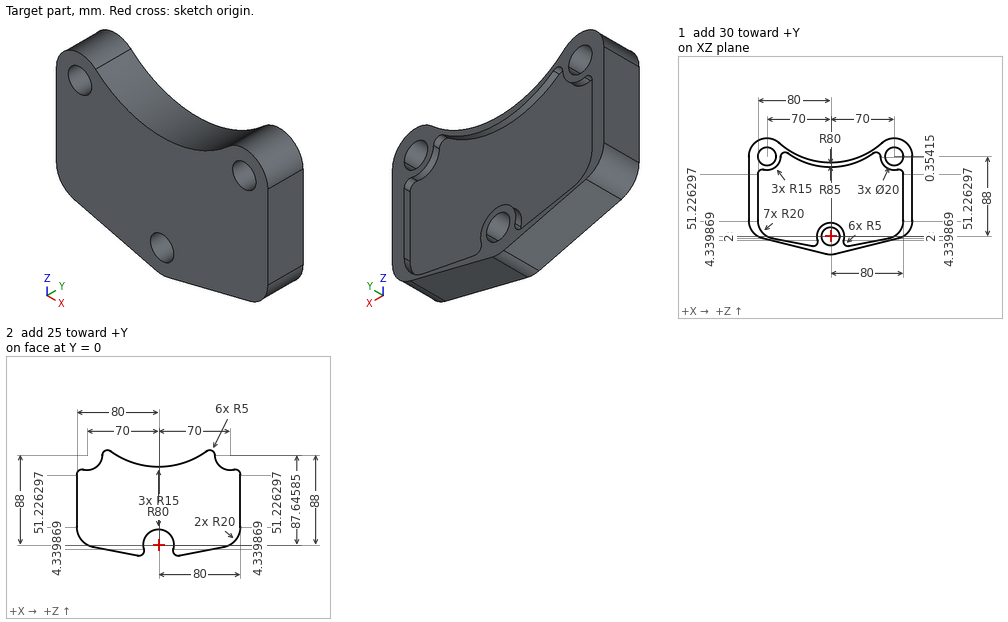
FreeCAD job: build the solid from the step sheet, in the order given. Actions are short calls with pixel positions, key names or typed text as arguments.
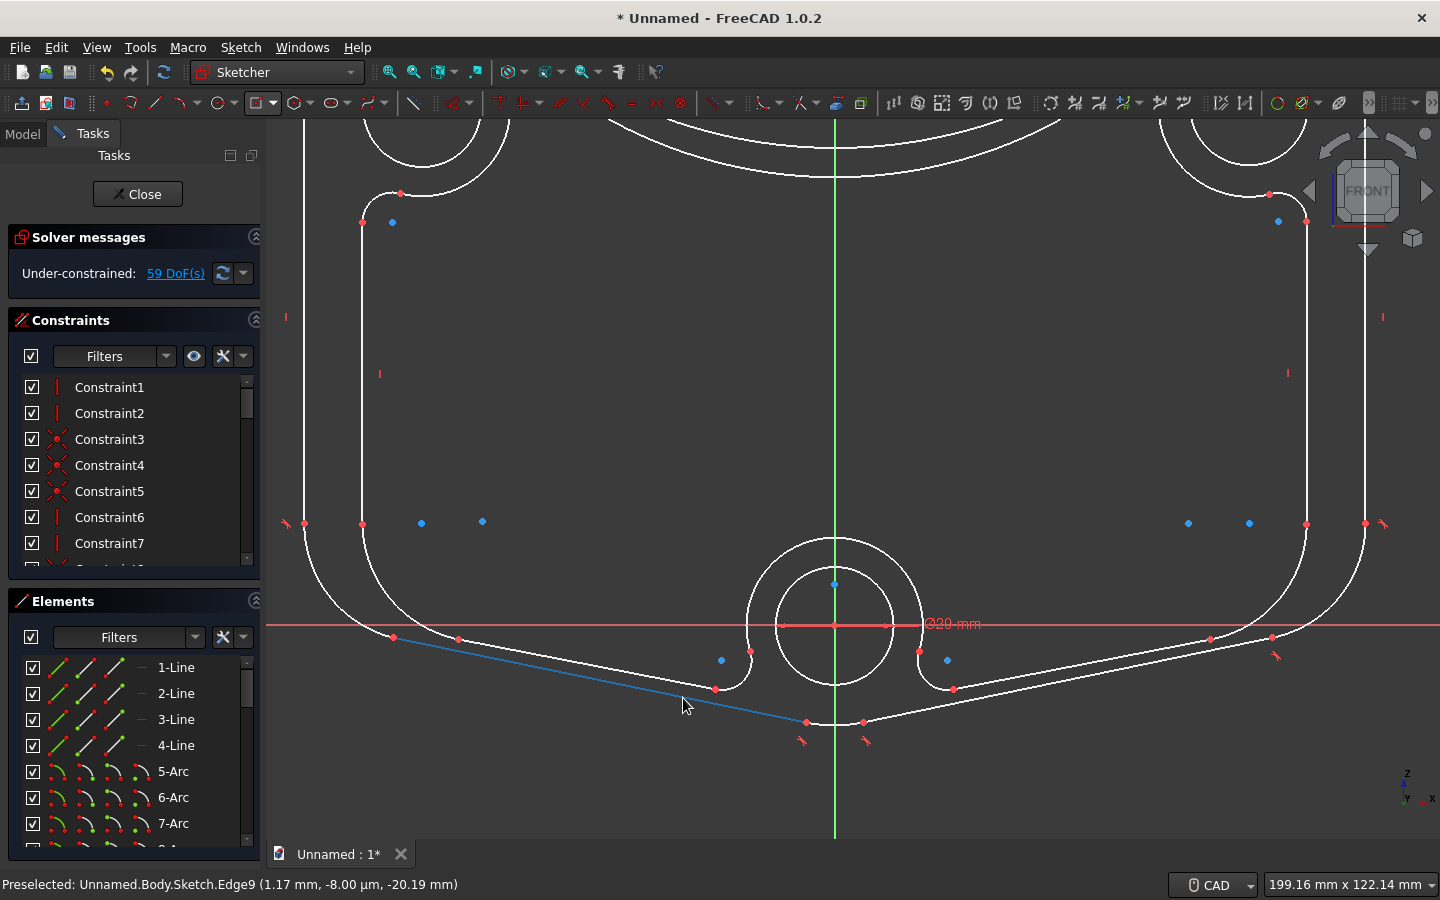
click(682, 697)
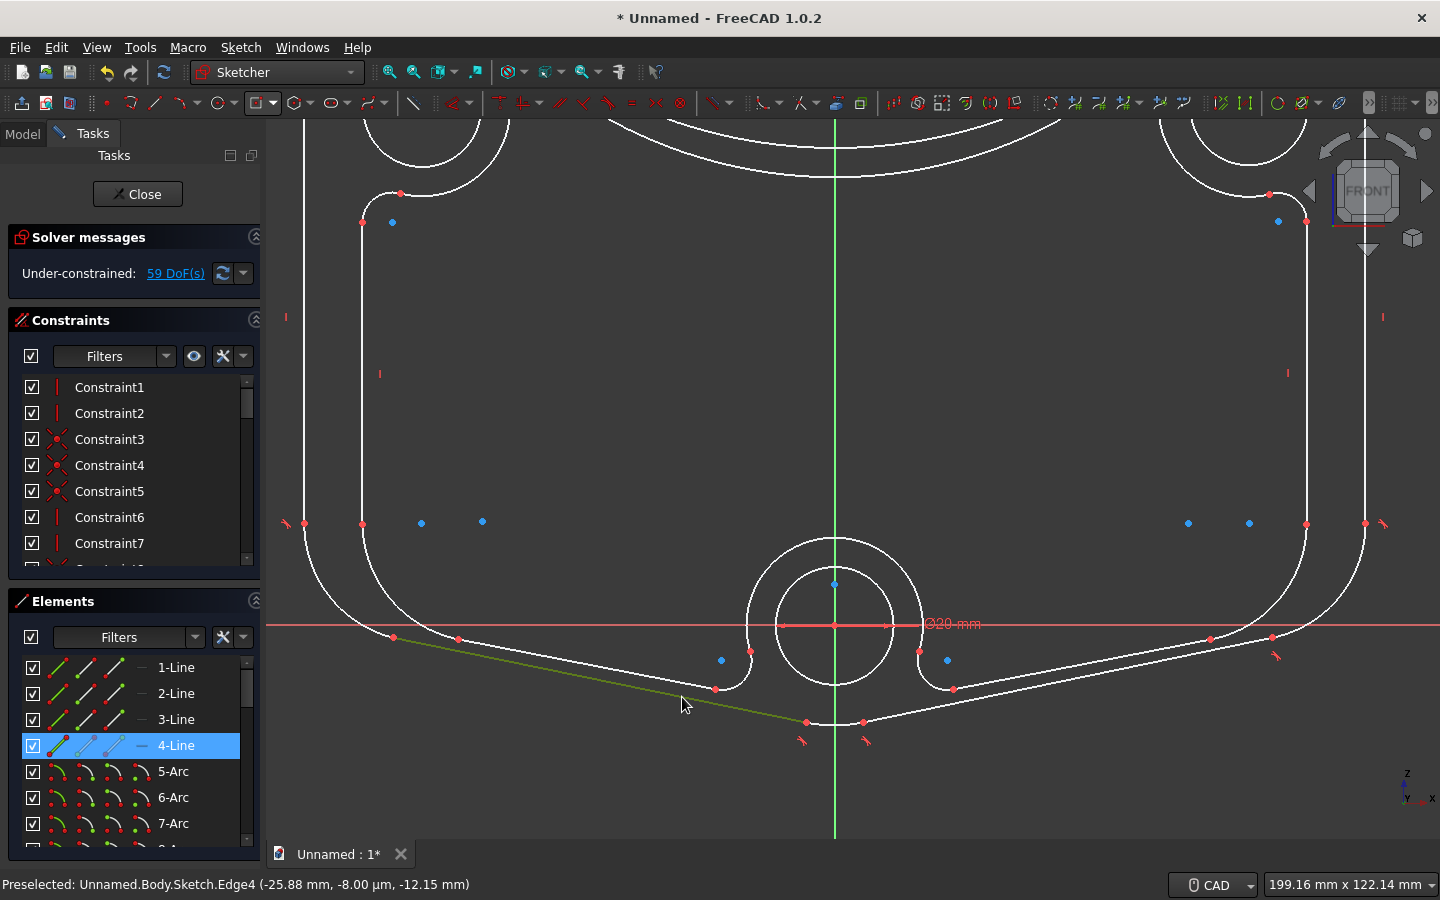
click(313, 569)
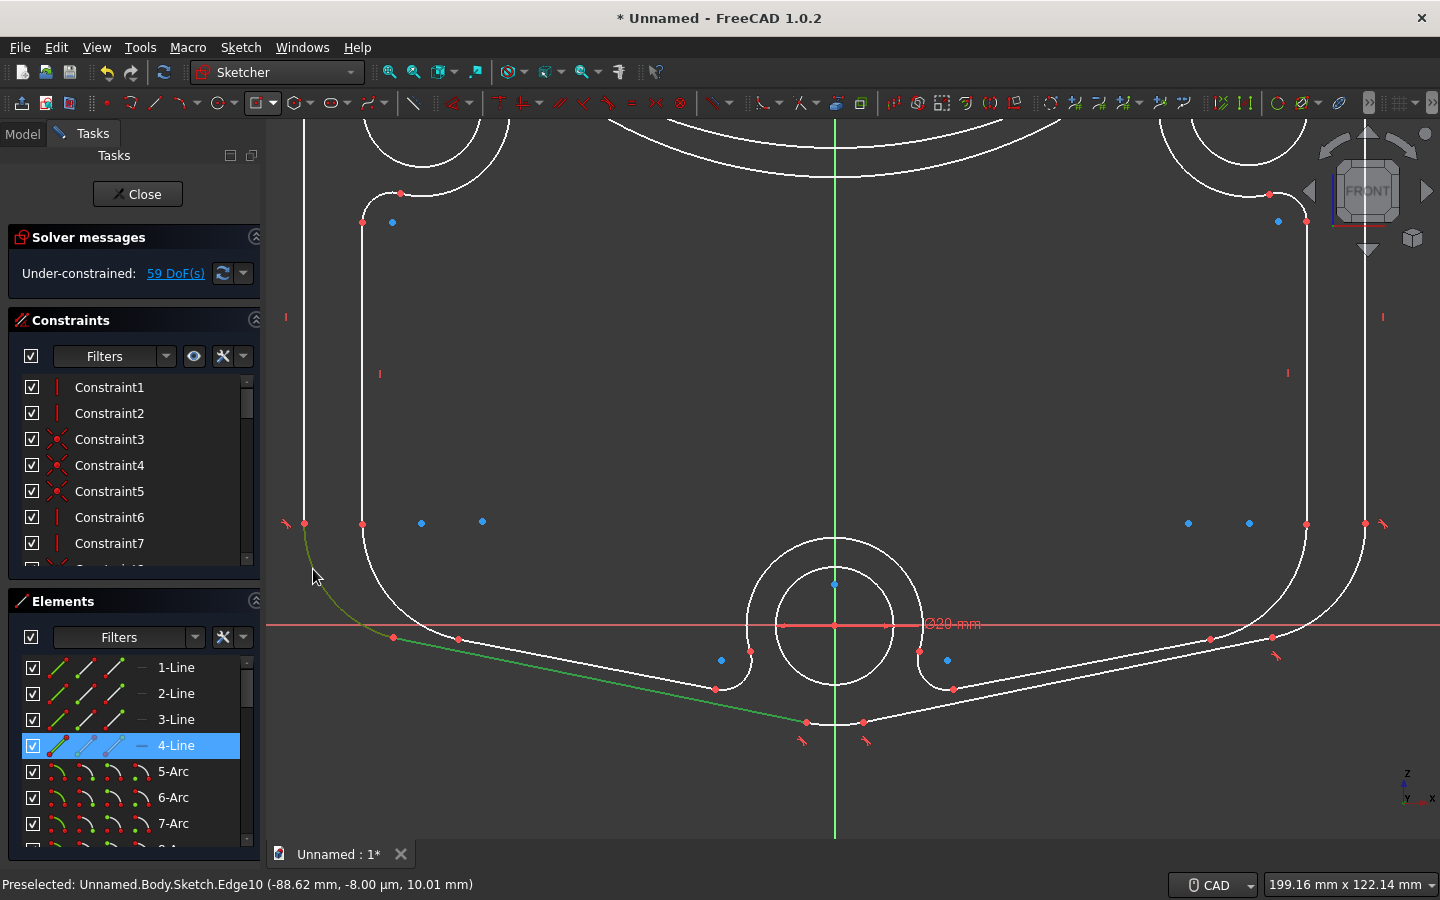
click(608, 104)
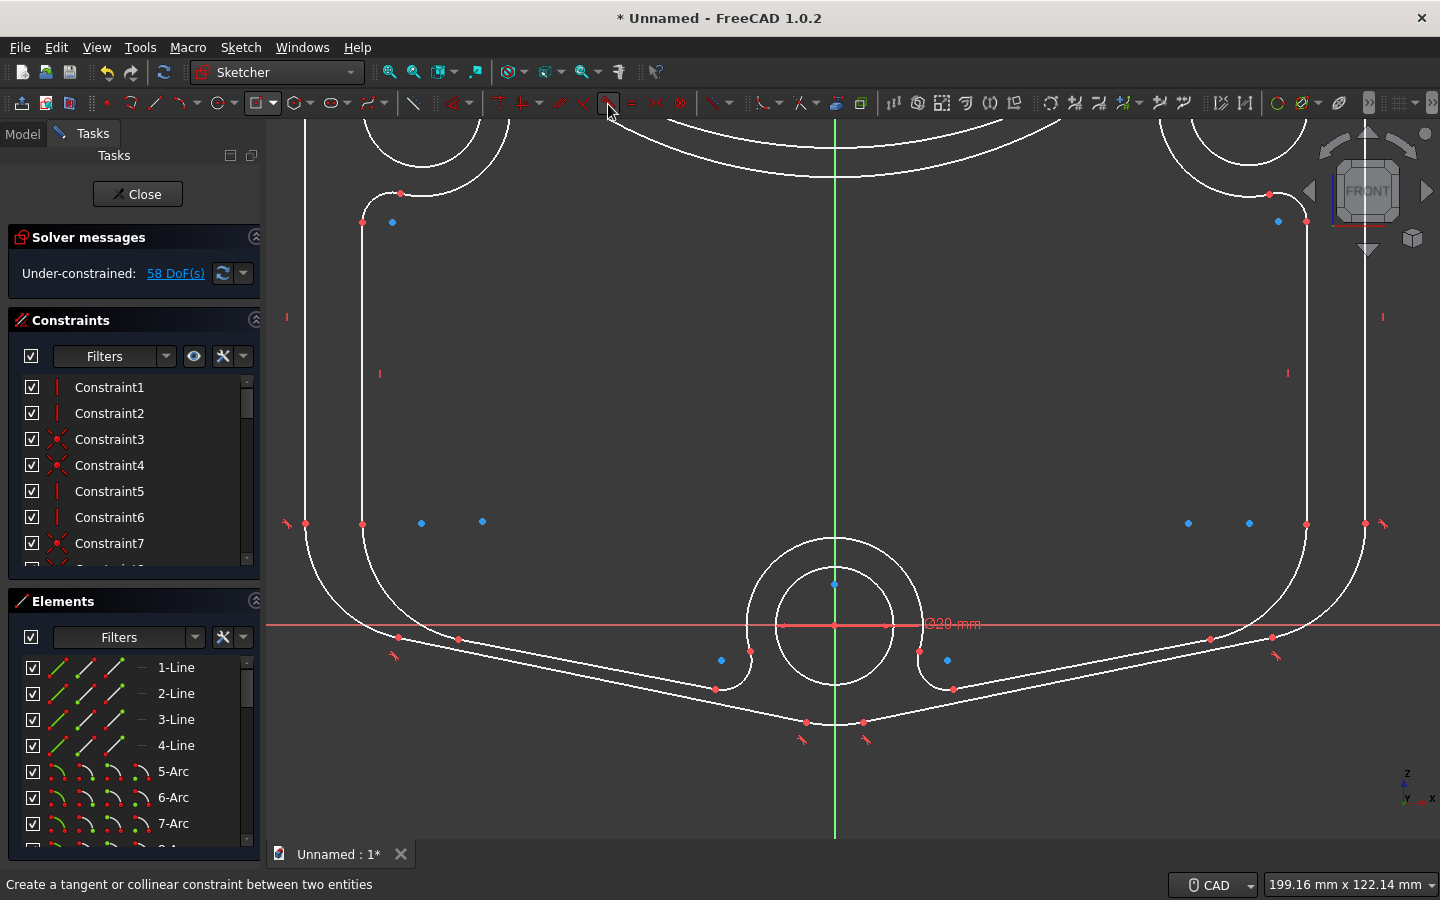
scroll(682, 698, down, 2)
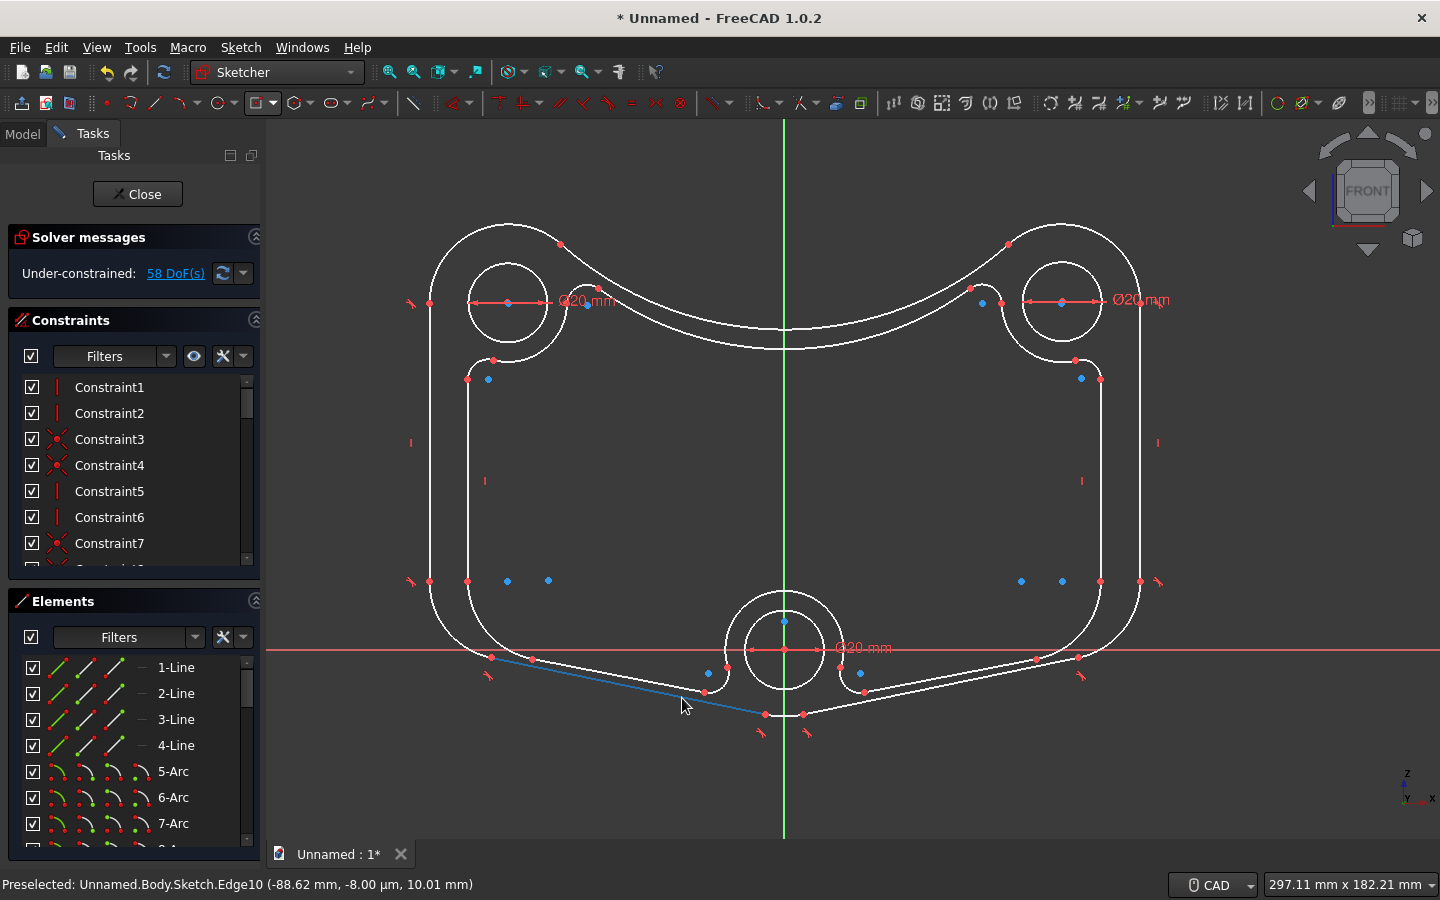
click(511, 224)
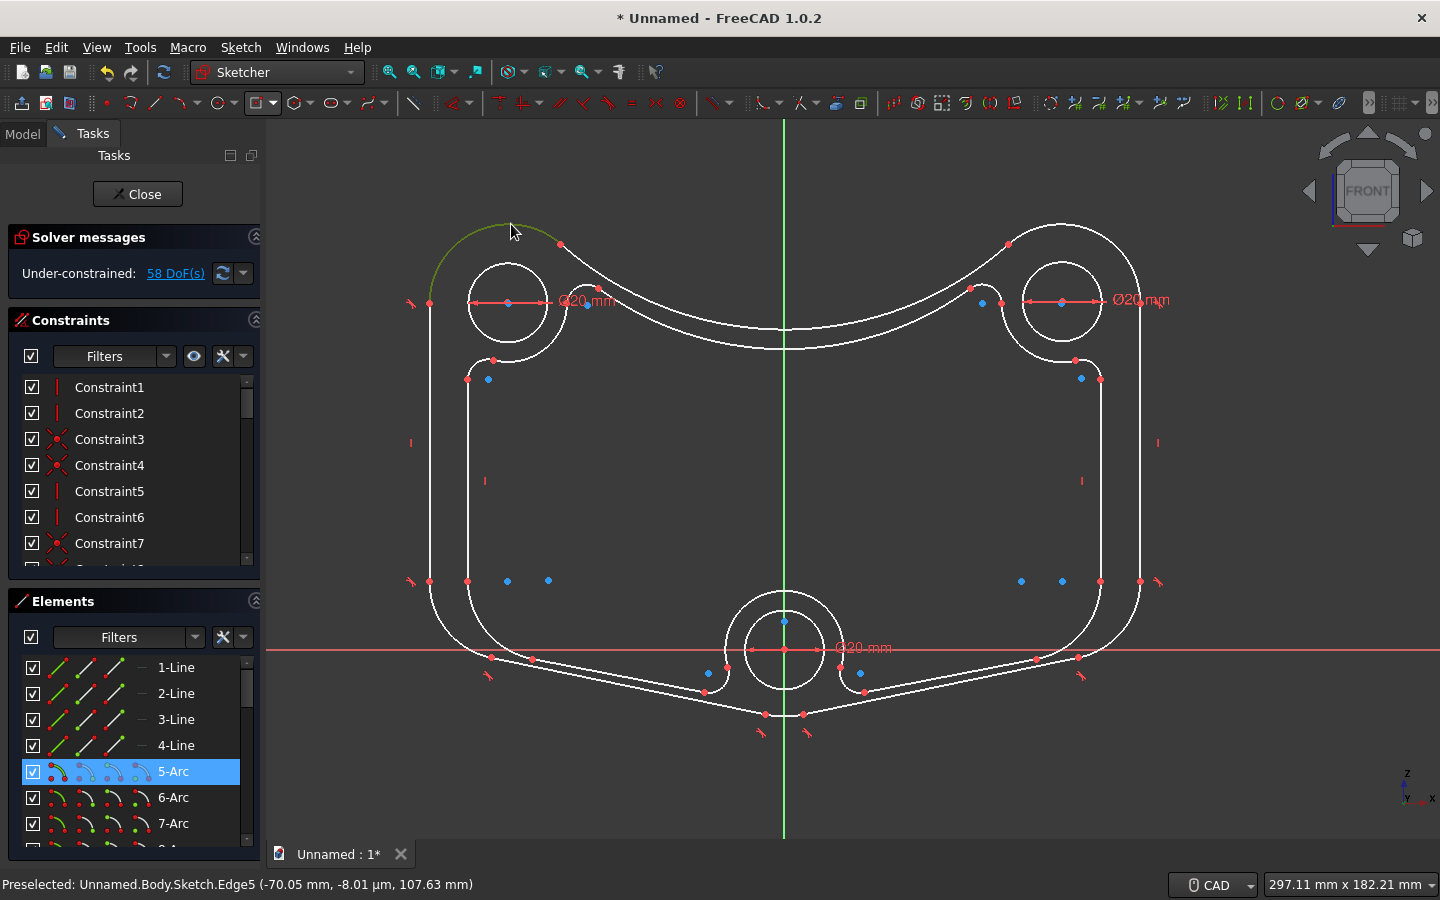
click(688, 315)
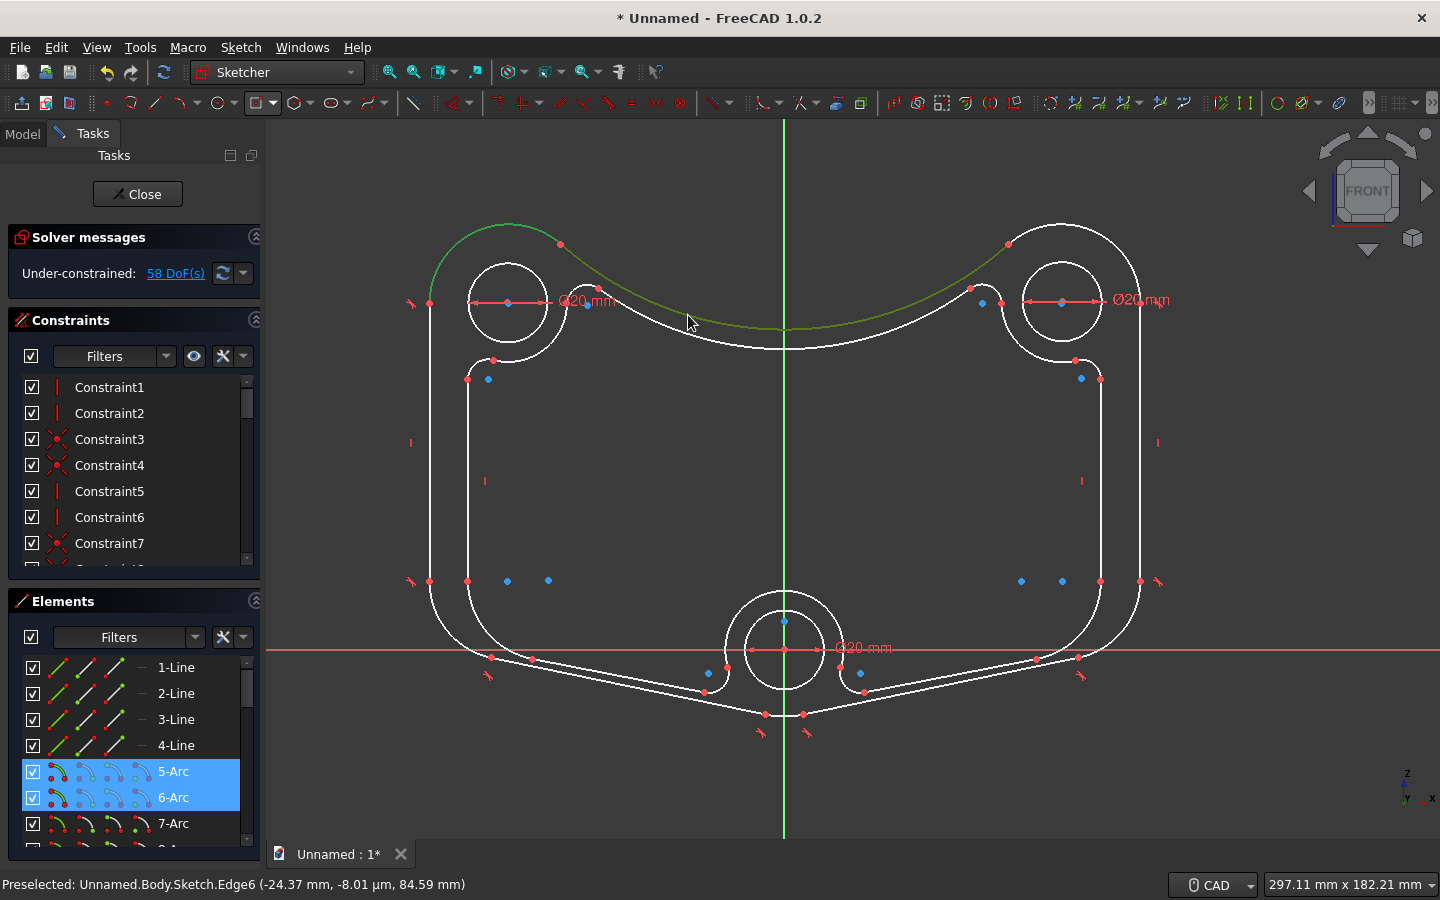
click(608, 104)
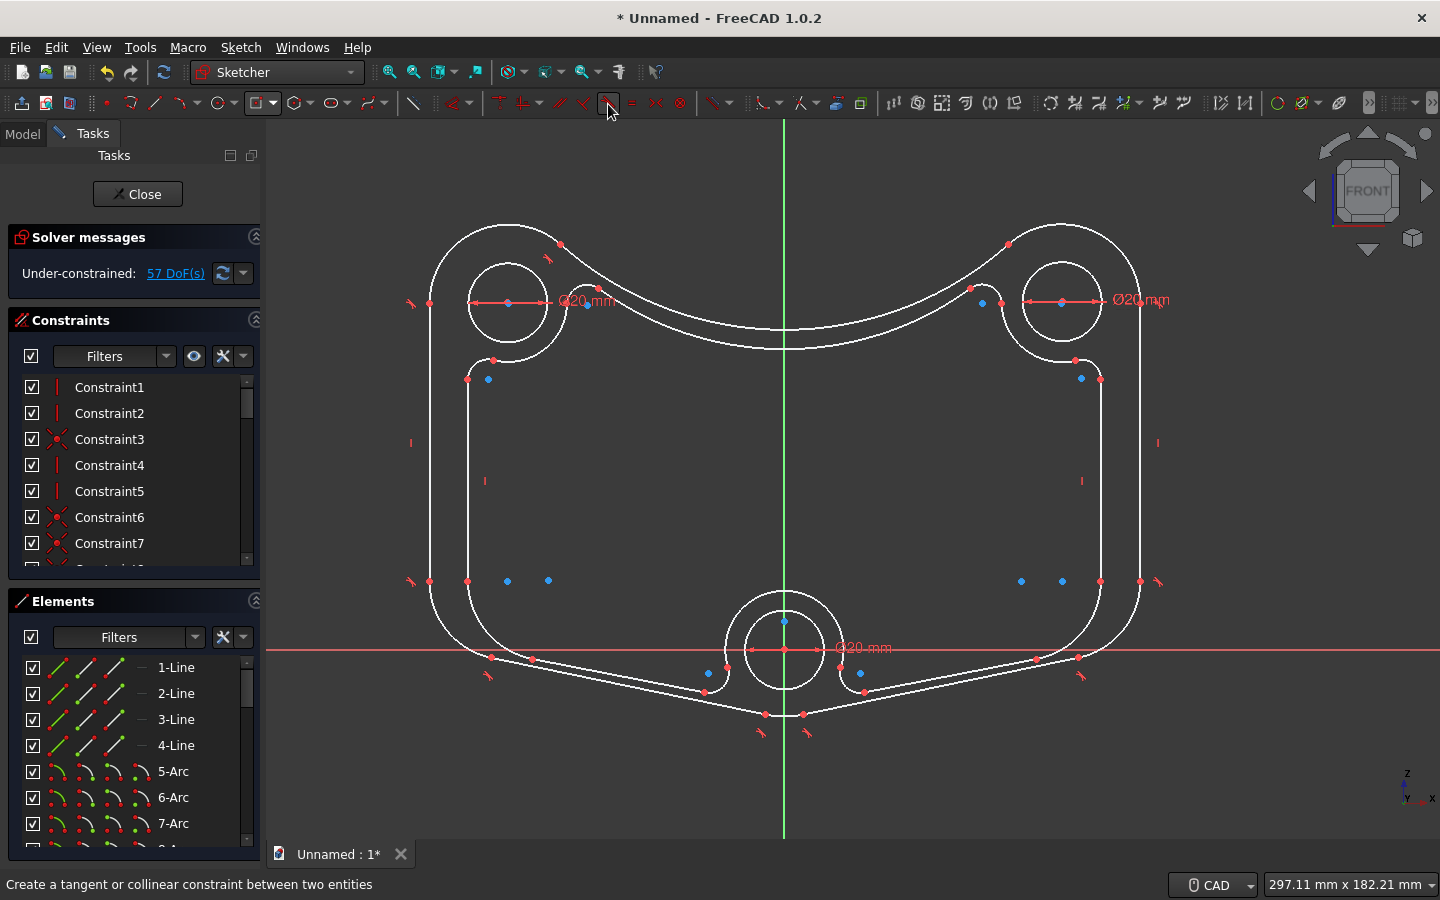
click(688, 316)